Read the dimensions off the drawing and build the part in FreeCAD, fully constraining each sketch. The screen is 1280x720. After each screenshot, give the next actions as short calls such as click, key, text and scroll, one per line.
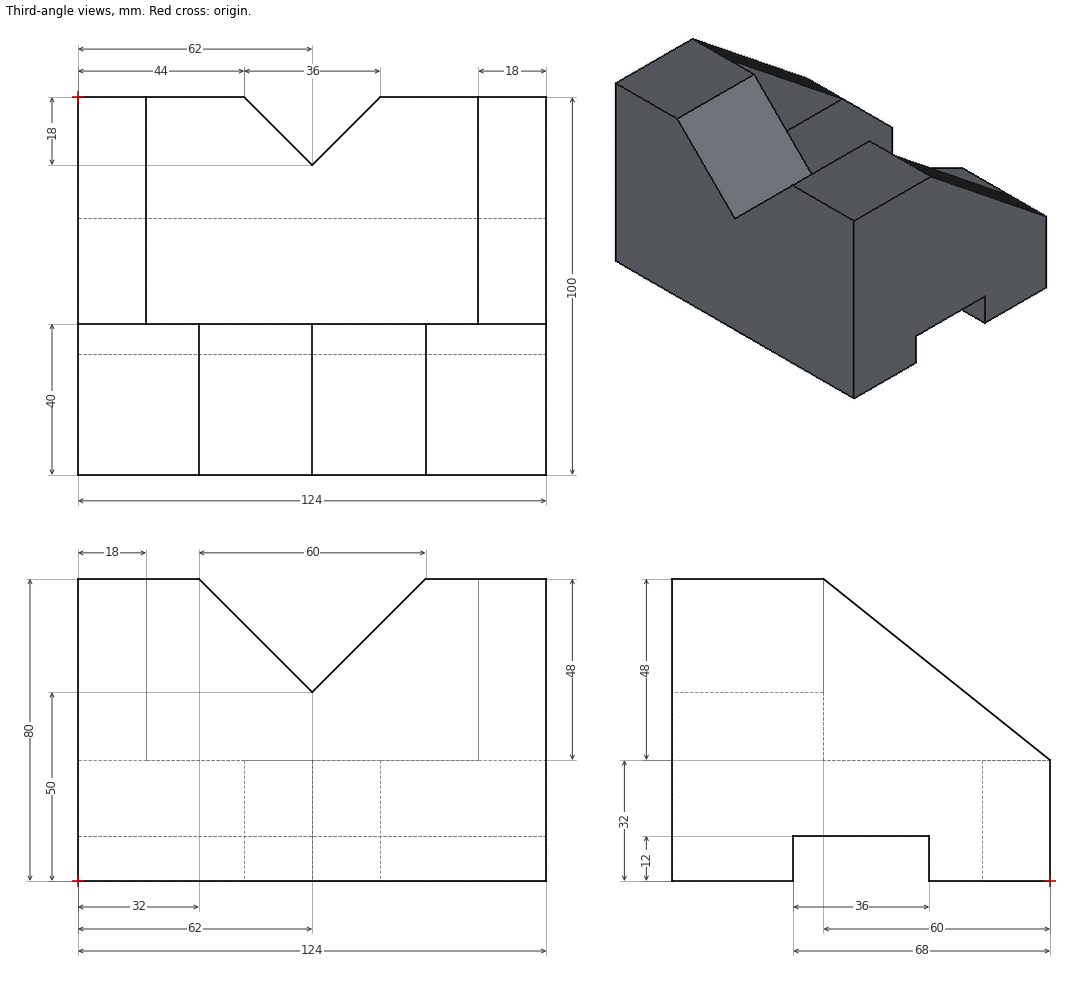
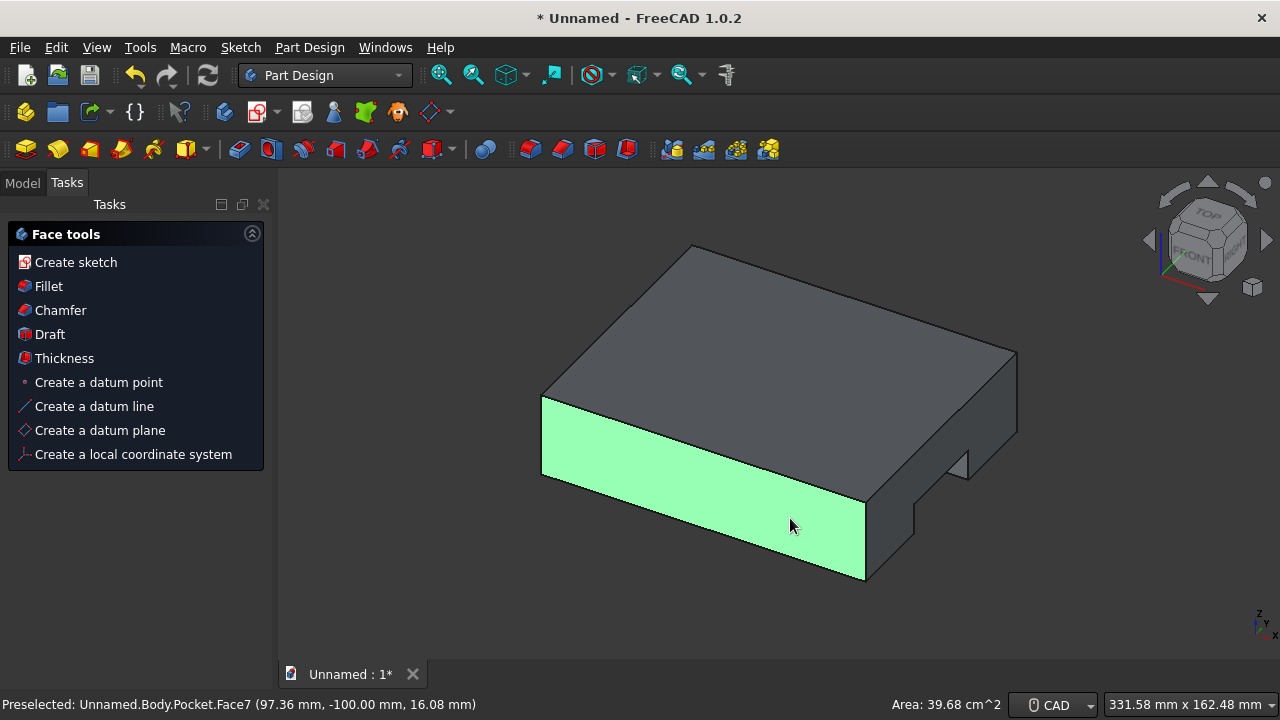
click(258, 112)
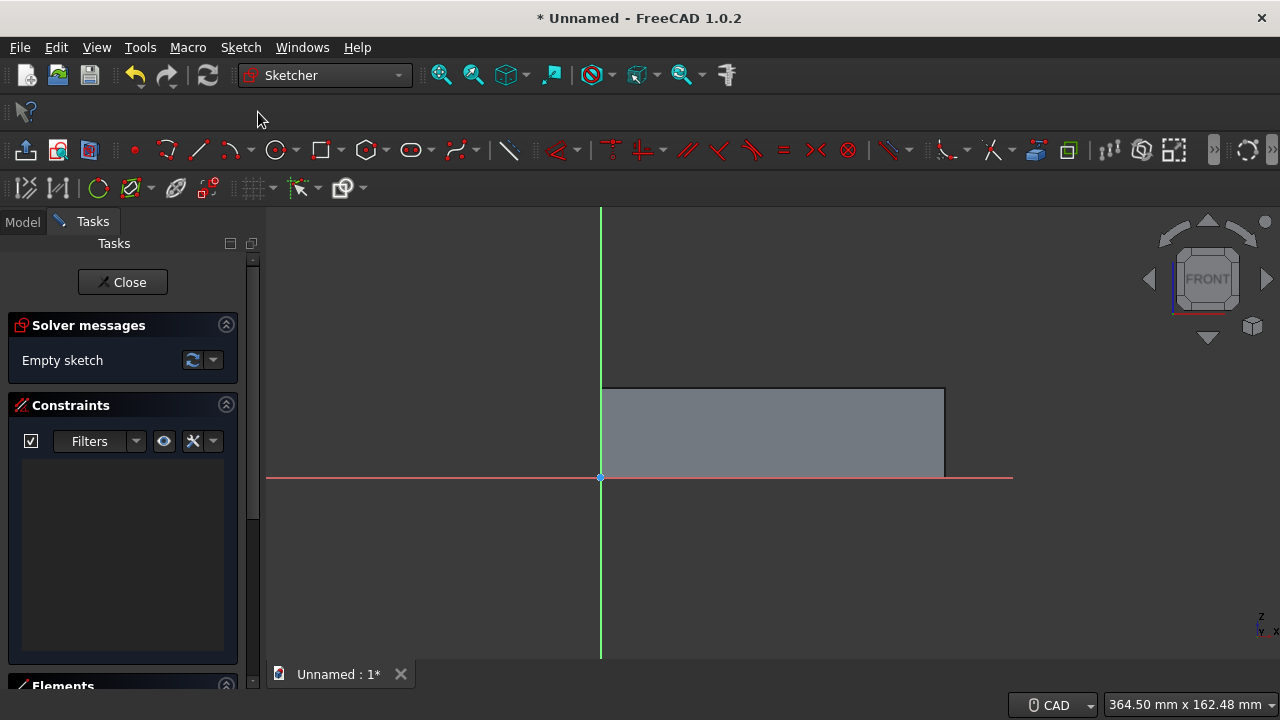
scroll(395, 631, down, 1)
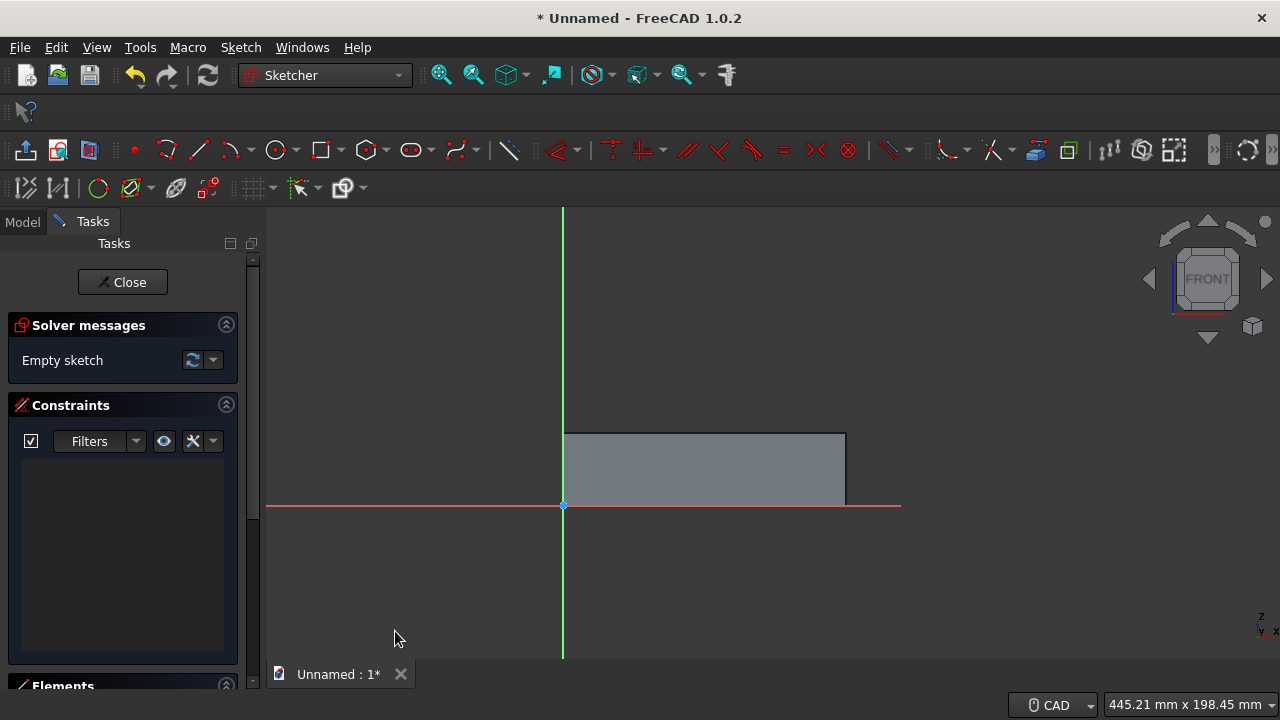
scroll(705, 377, up, 2)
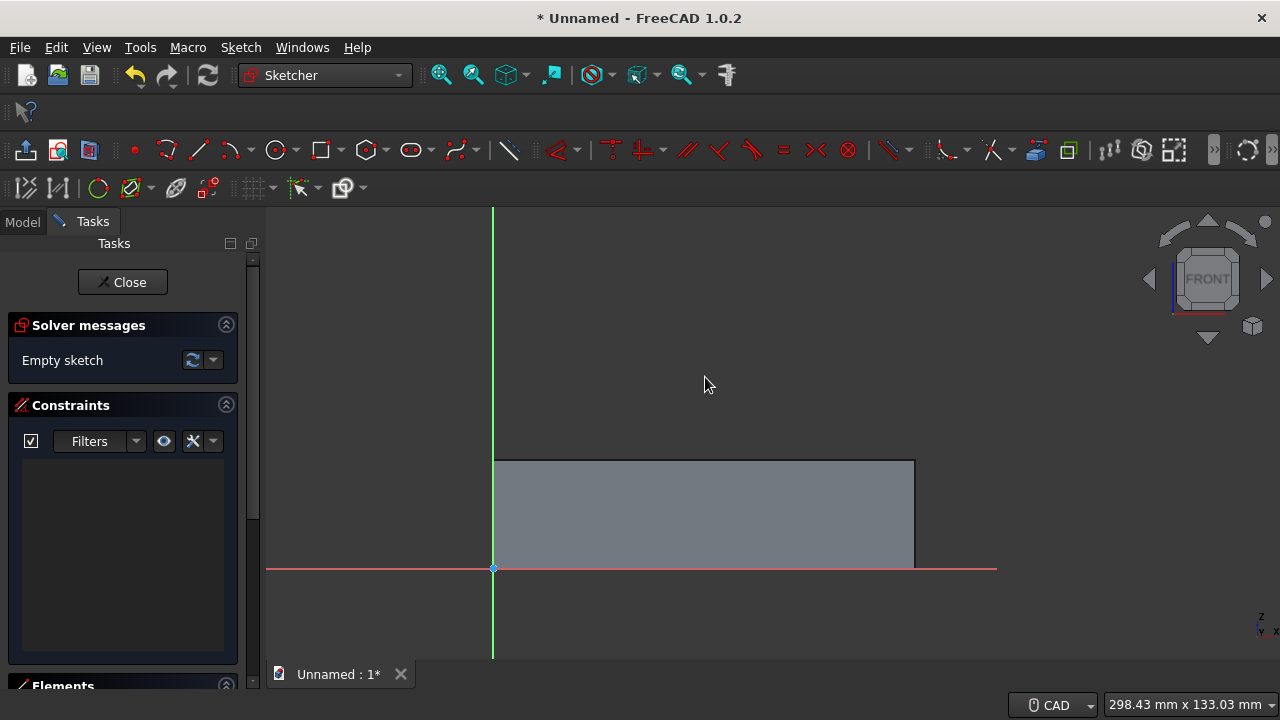
click(322, 150)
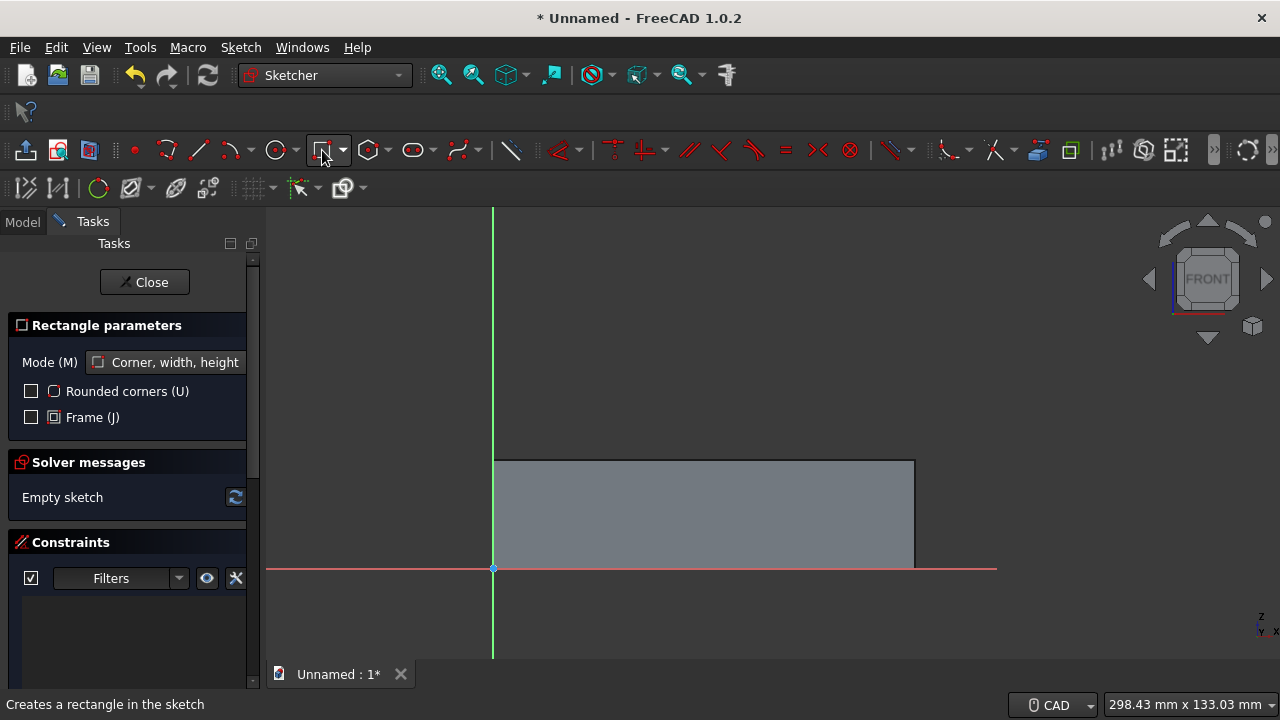
click(493, 297)
move(915, 460)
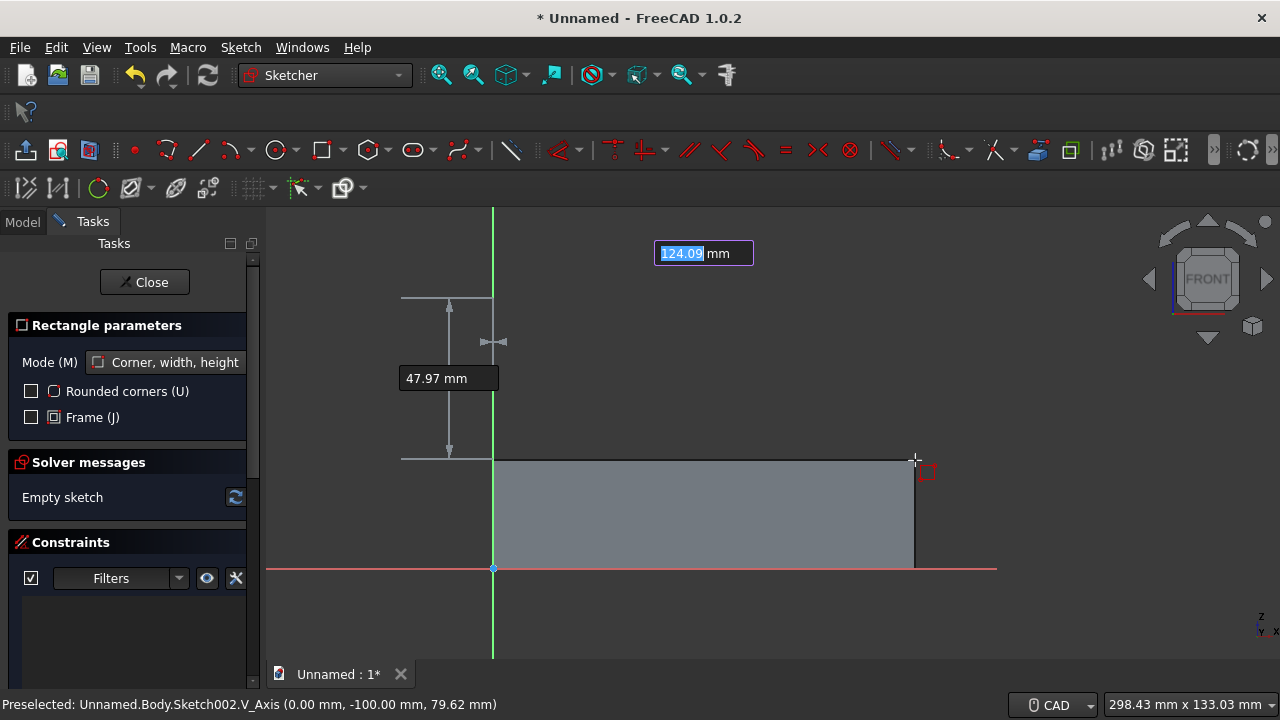
text(124)
key(Tab)
text(48)
key(Return)
key(Escape)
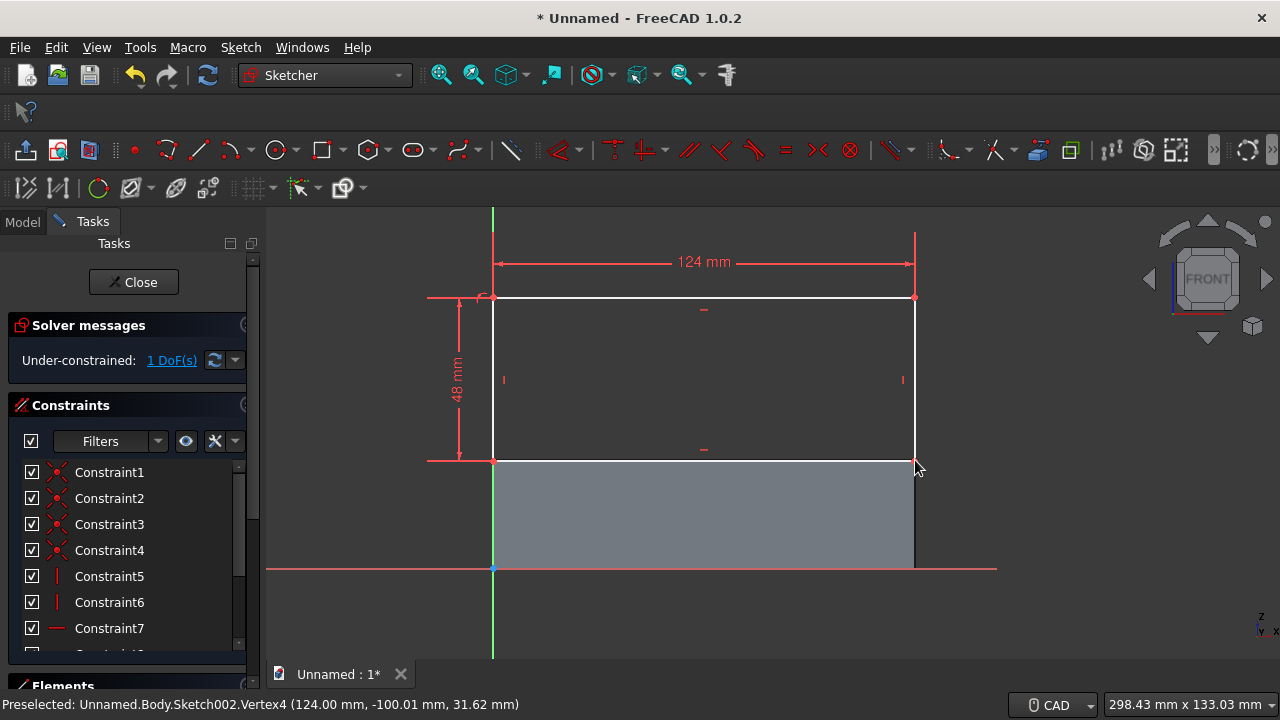
click(558, 150)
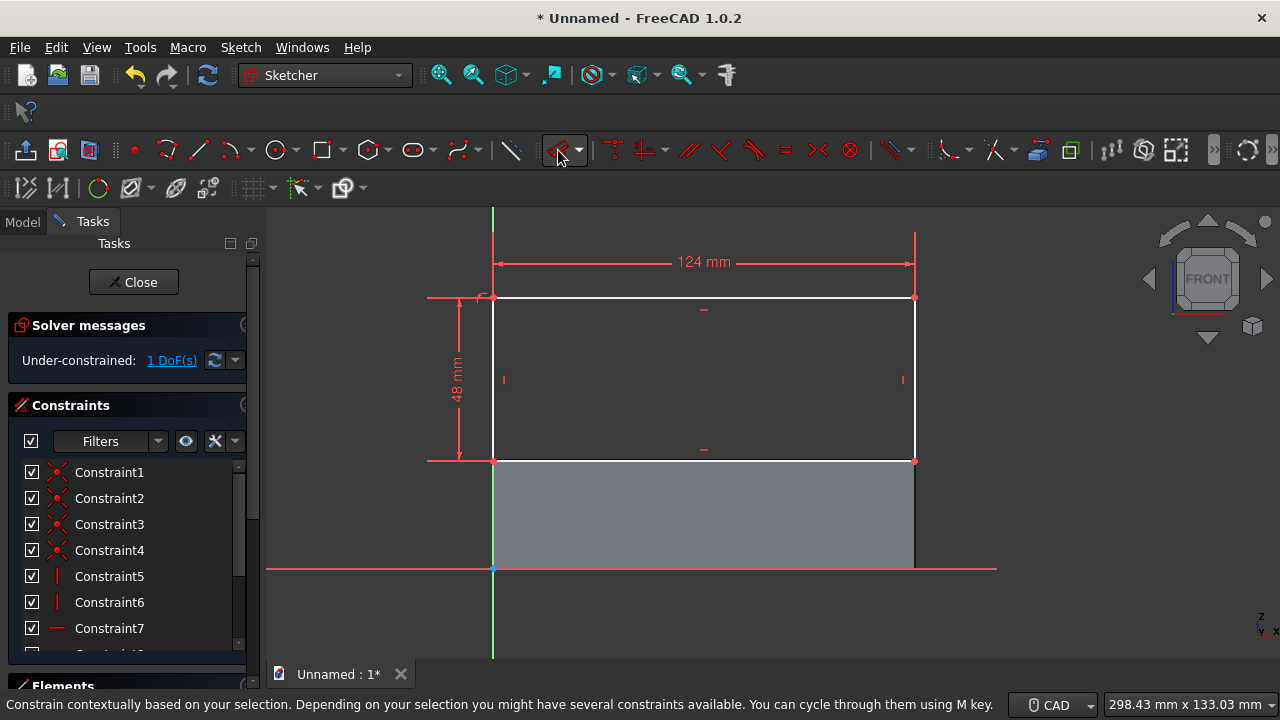
click(493, 298)
click(459, 433)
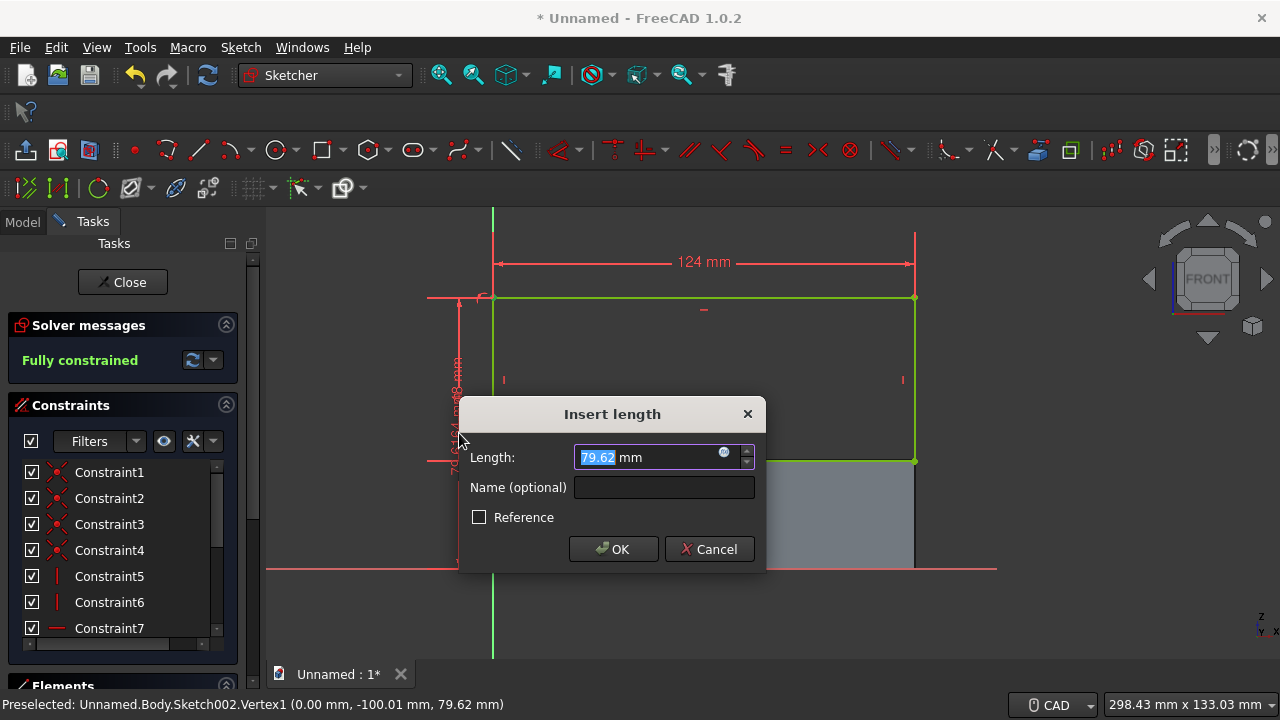
text(80)
key(Return)
key(Escape)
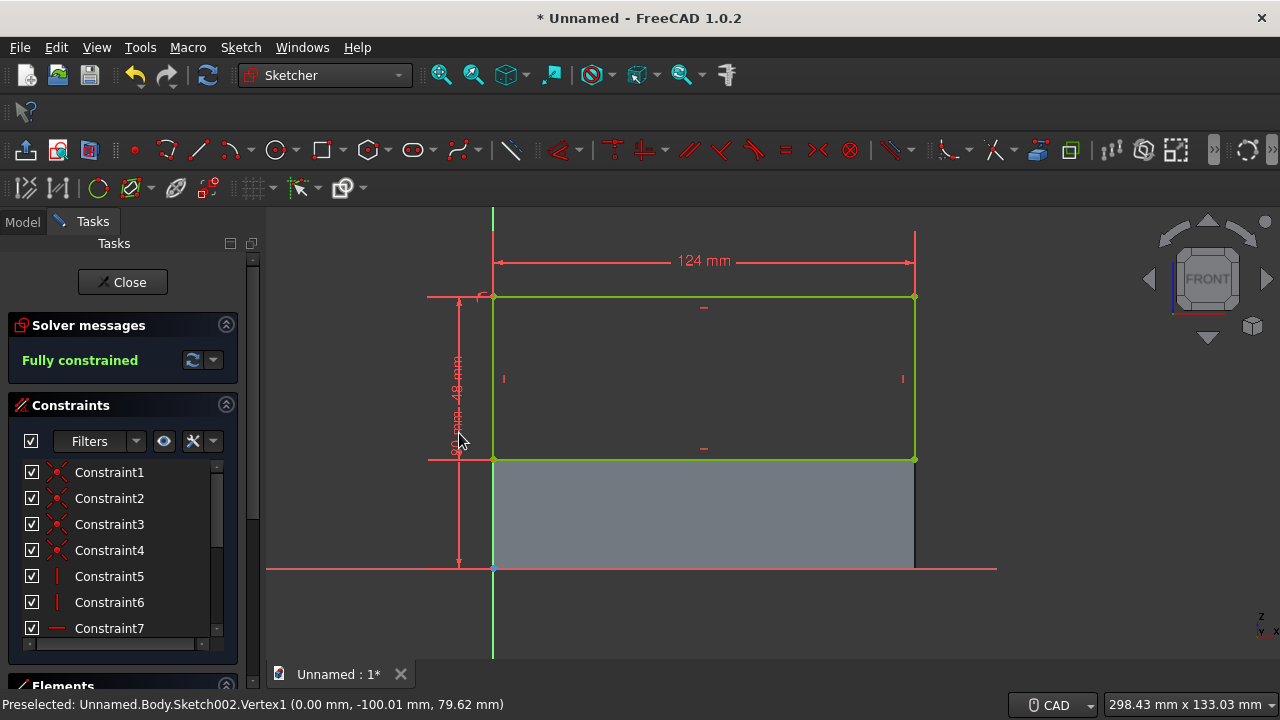
click(123, 282)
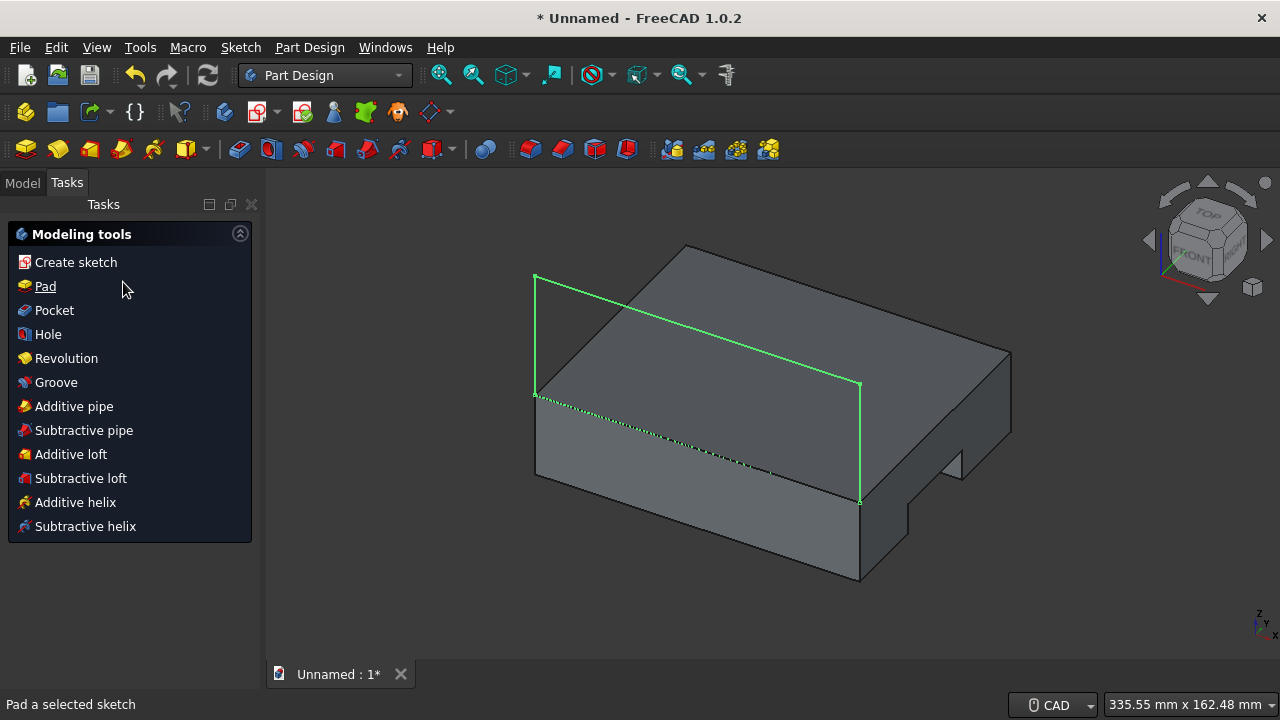
click(26, 150)